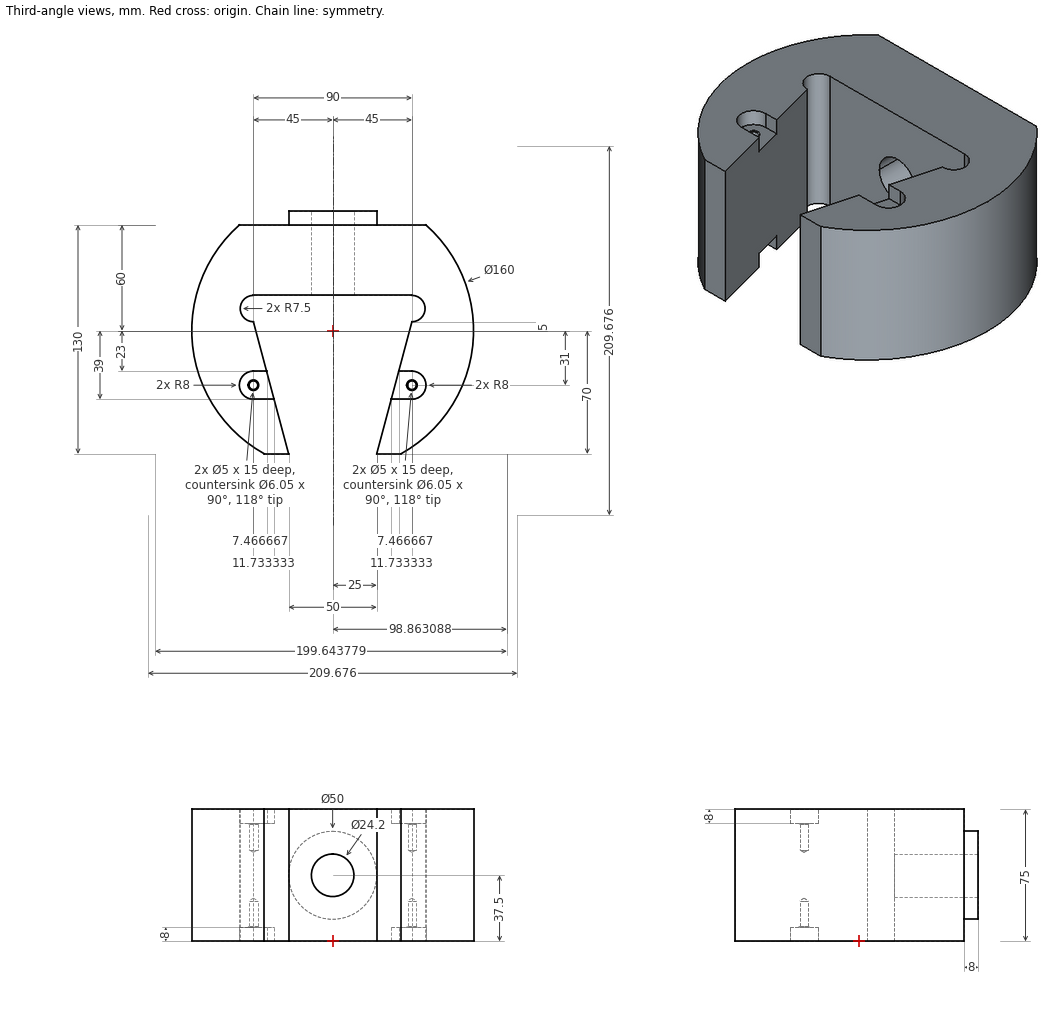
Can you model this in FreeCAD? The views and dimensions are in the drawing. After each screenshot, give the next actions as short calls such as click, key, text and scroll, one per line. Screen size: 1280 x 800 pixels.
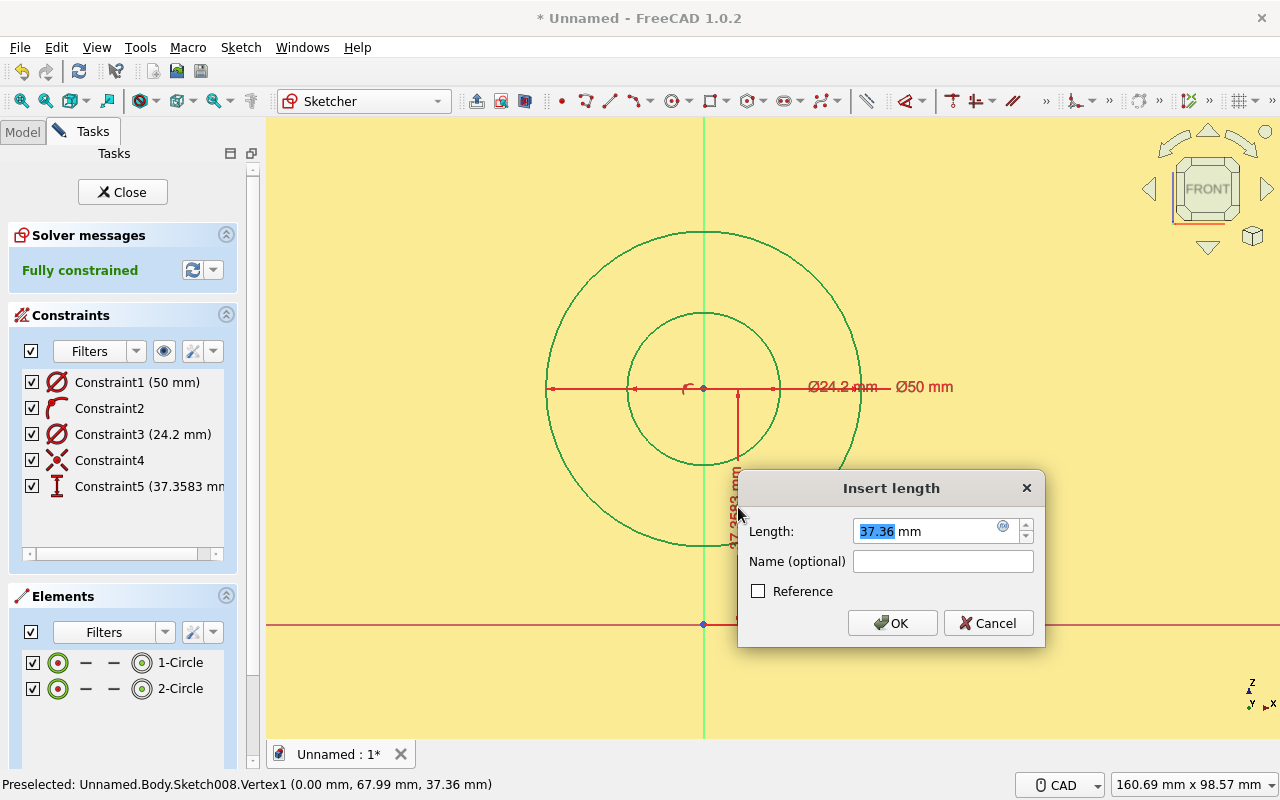
text(37.5)
key(Return)
key(Escape)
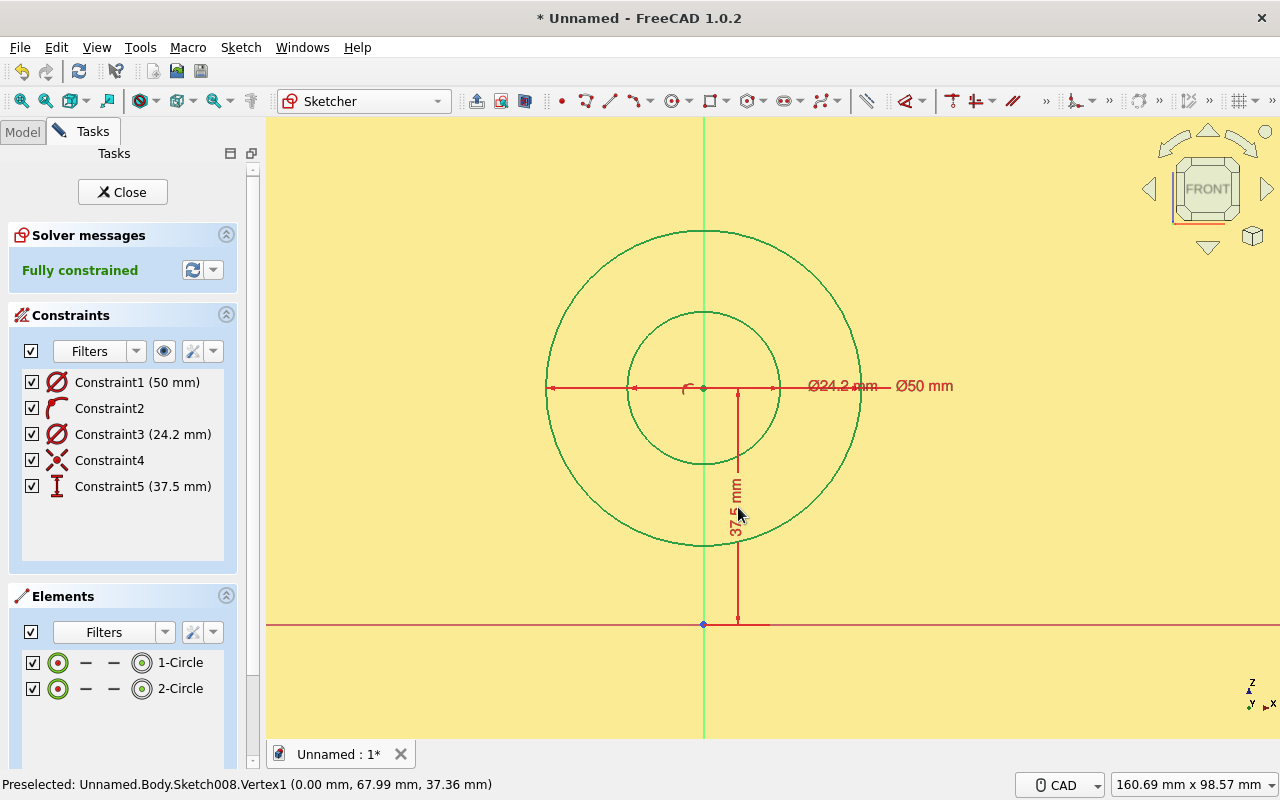
click(123, 192)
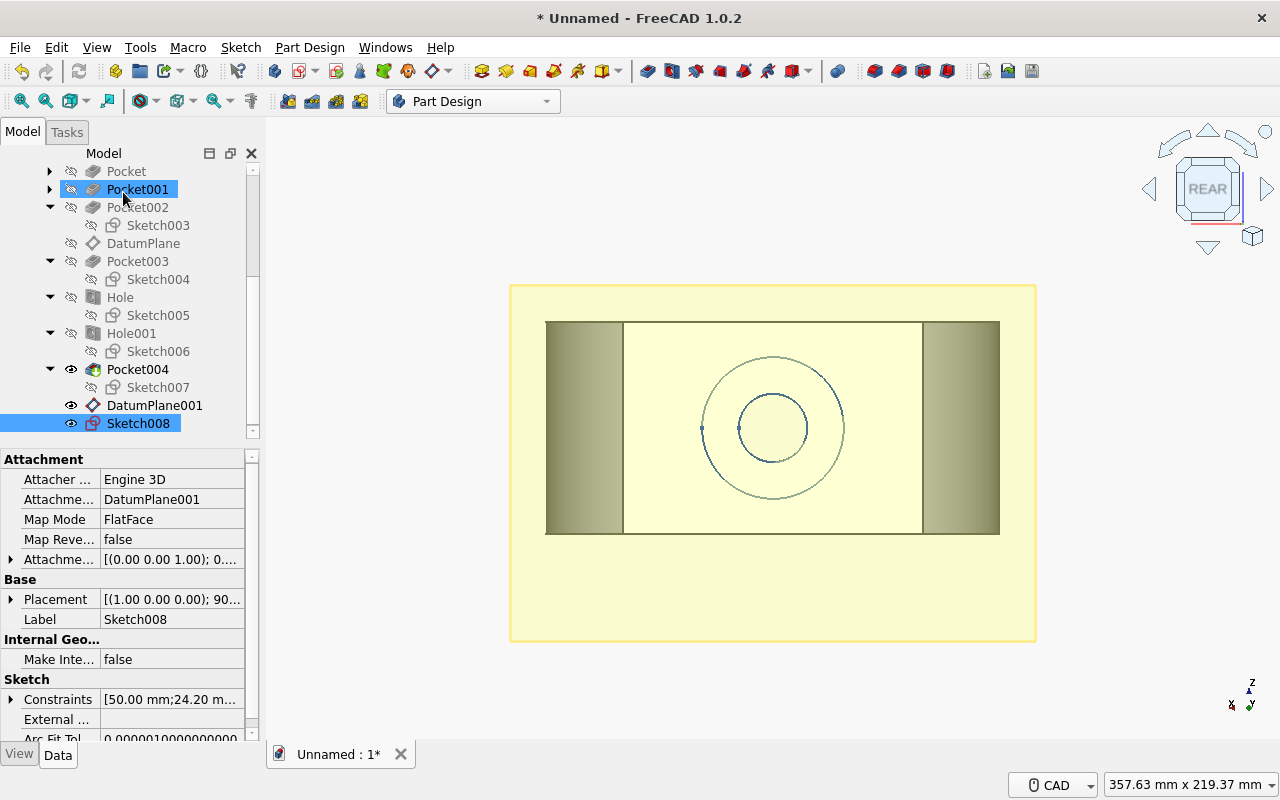
click(482, 72)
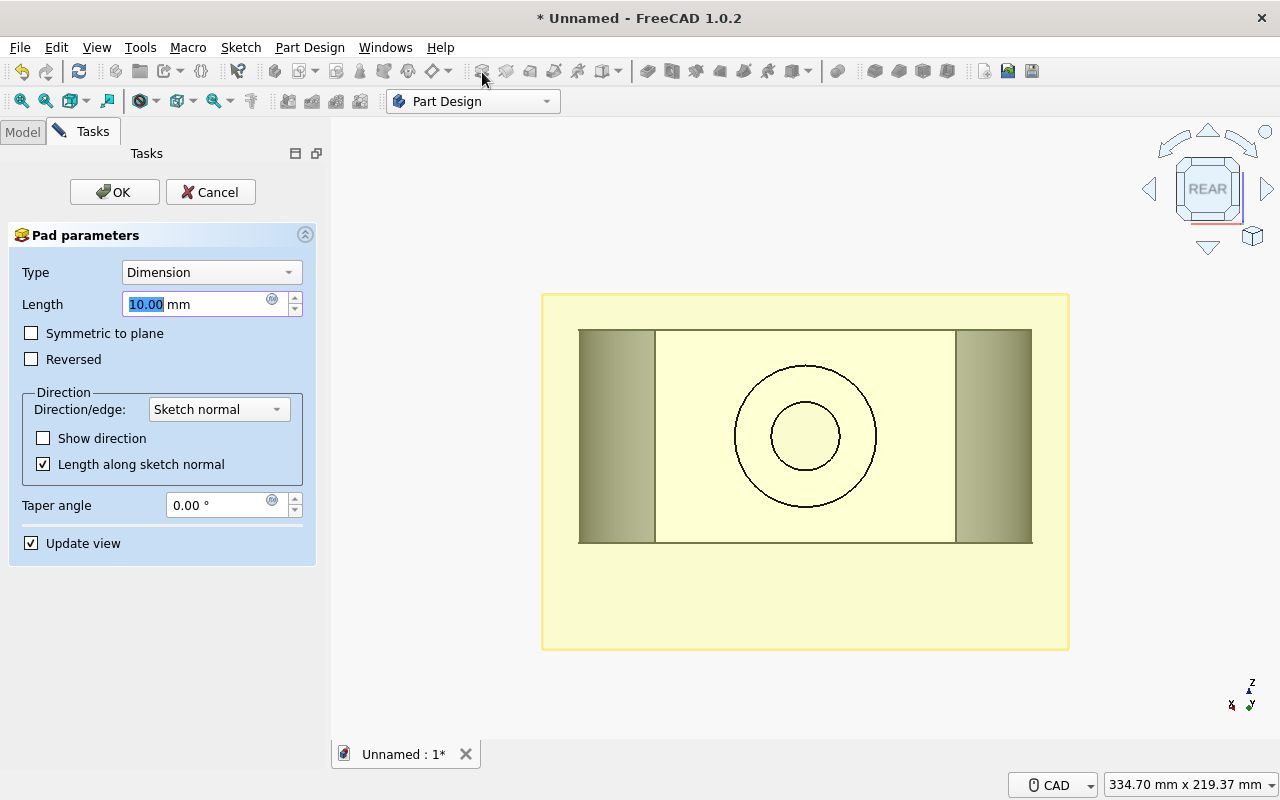
text(8)
key(Tab)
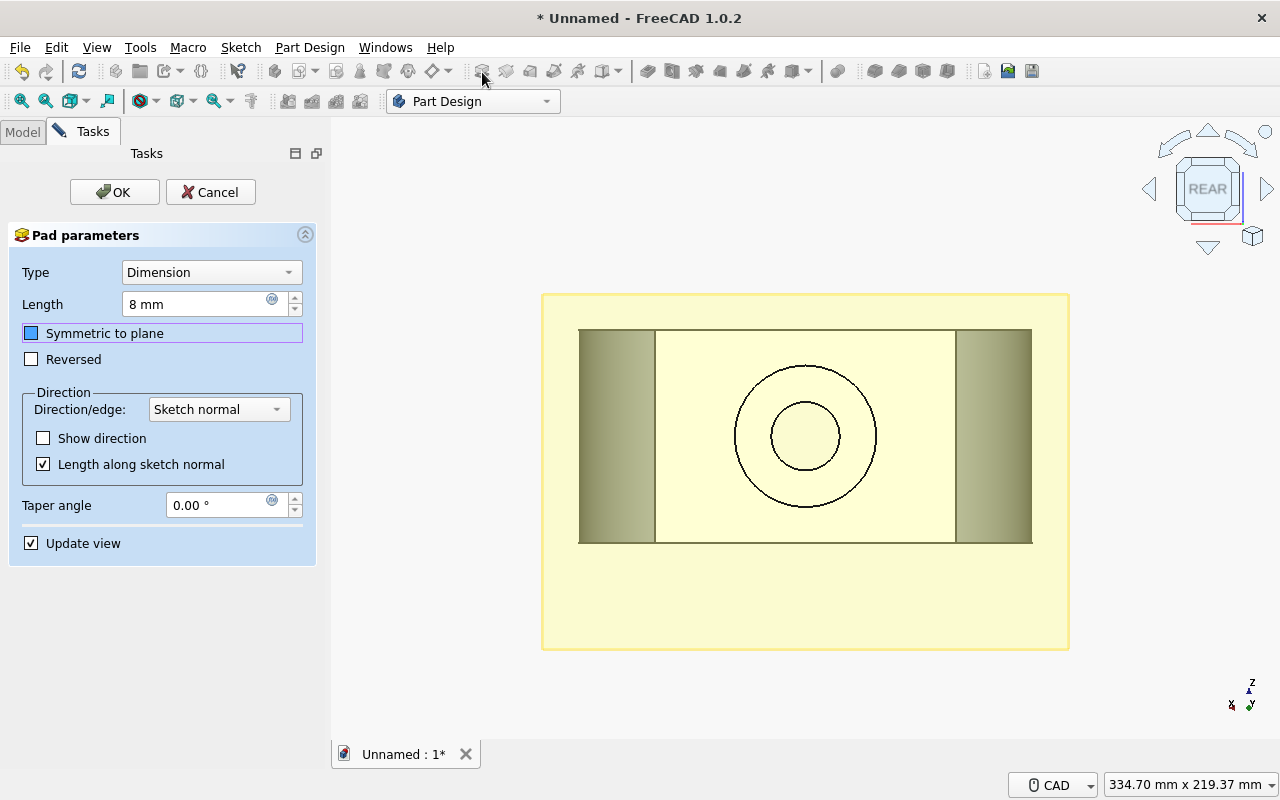
click(115, 192)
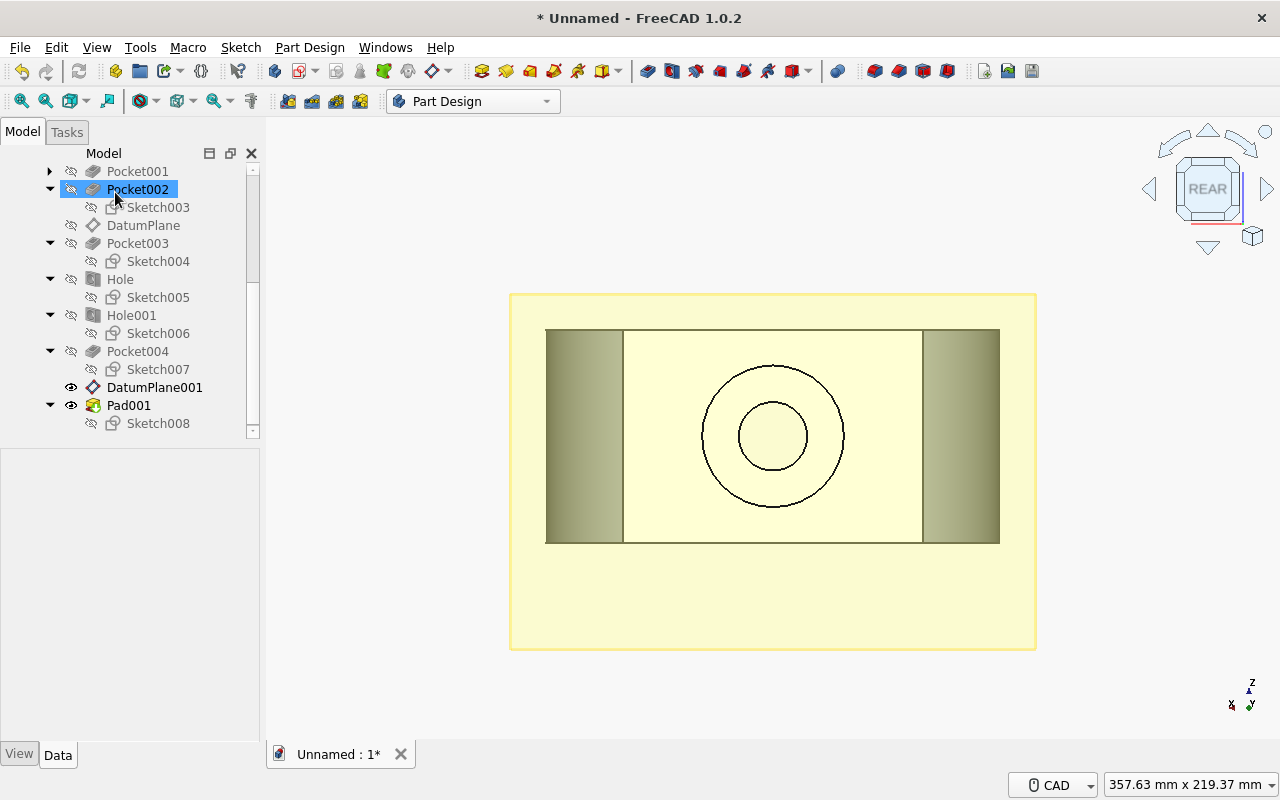
click(116, 387)
key(space)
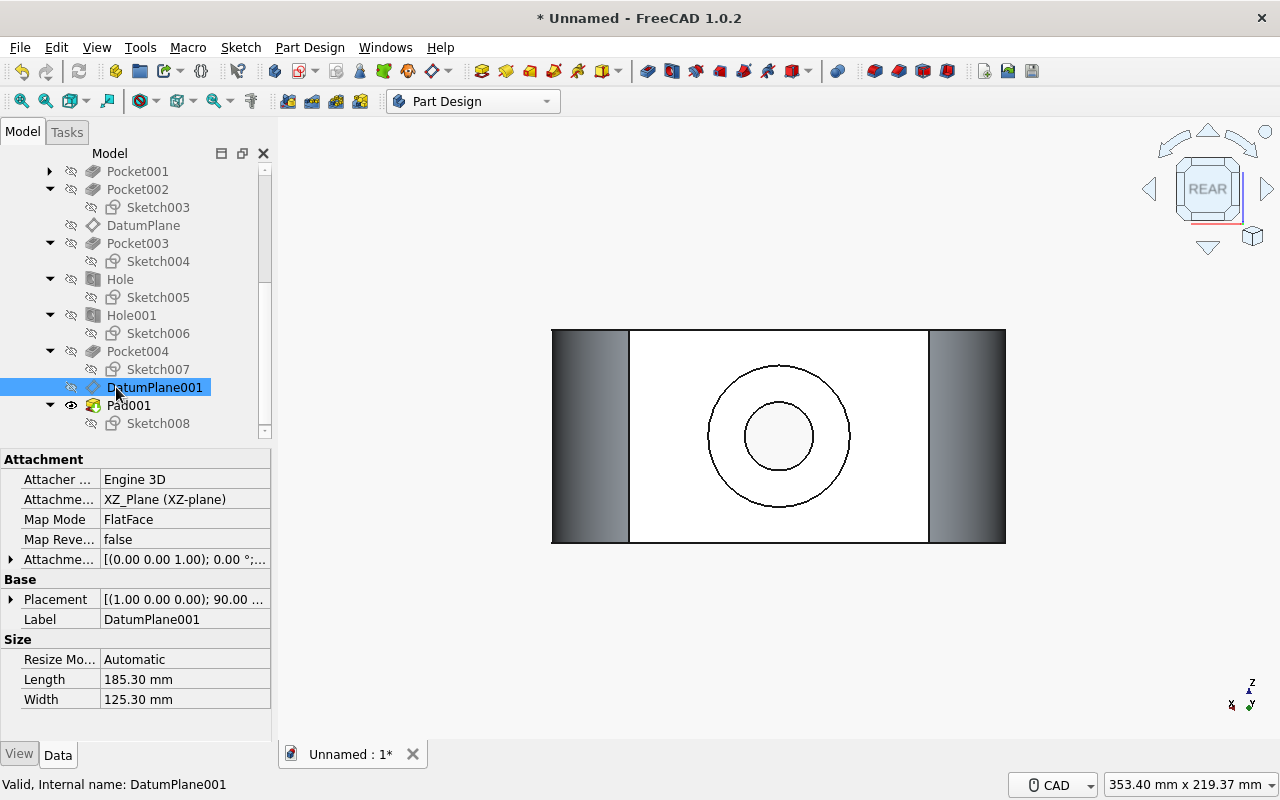
key(0)